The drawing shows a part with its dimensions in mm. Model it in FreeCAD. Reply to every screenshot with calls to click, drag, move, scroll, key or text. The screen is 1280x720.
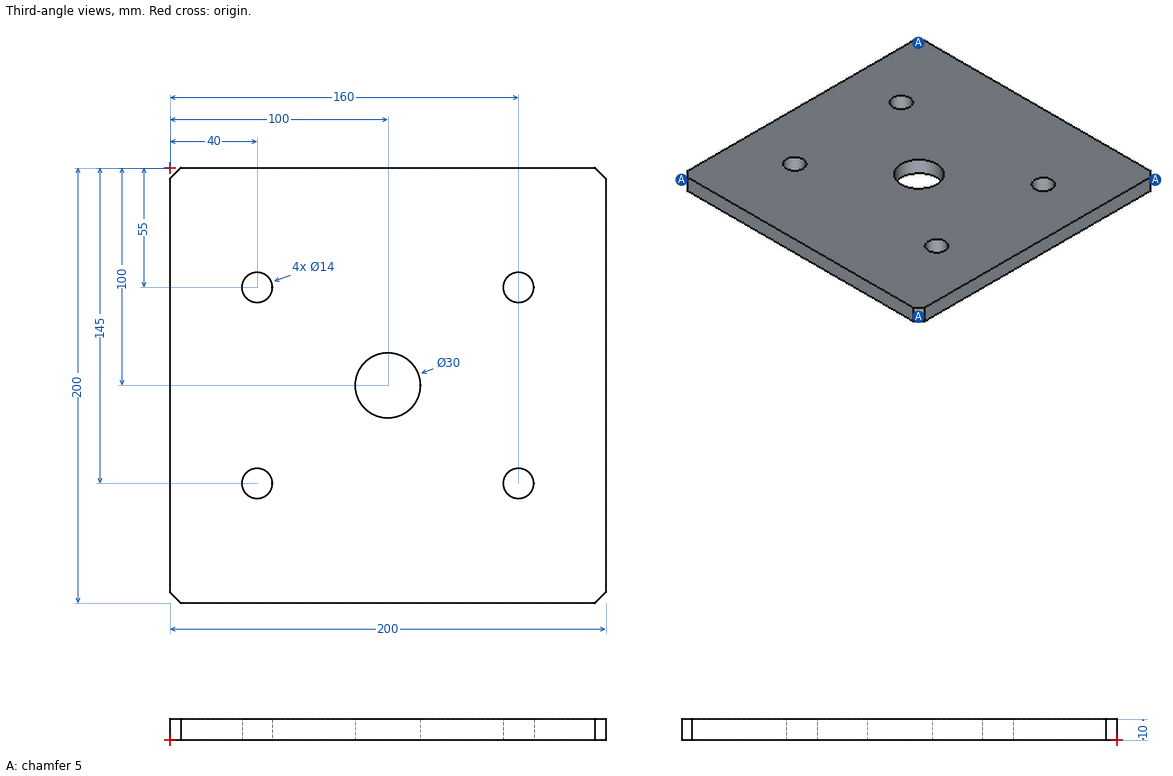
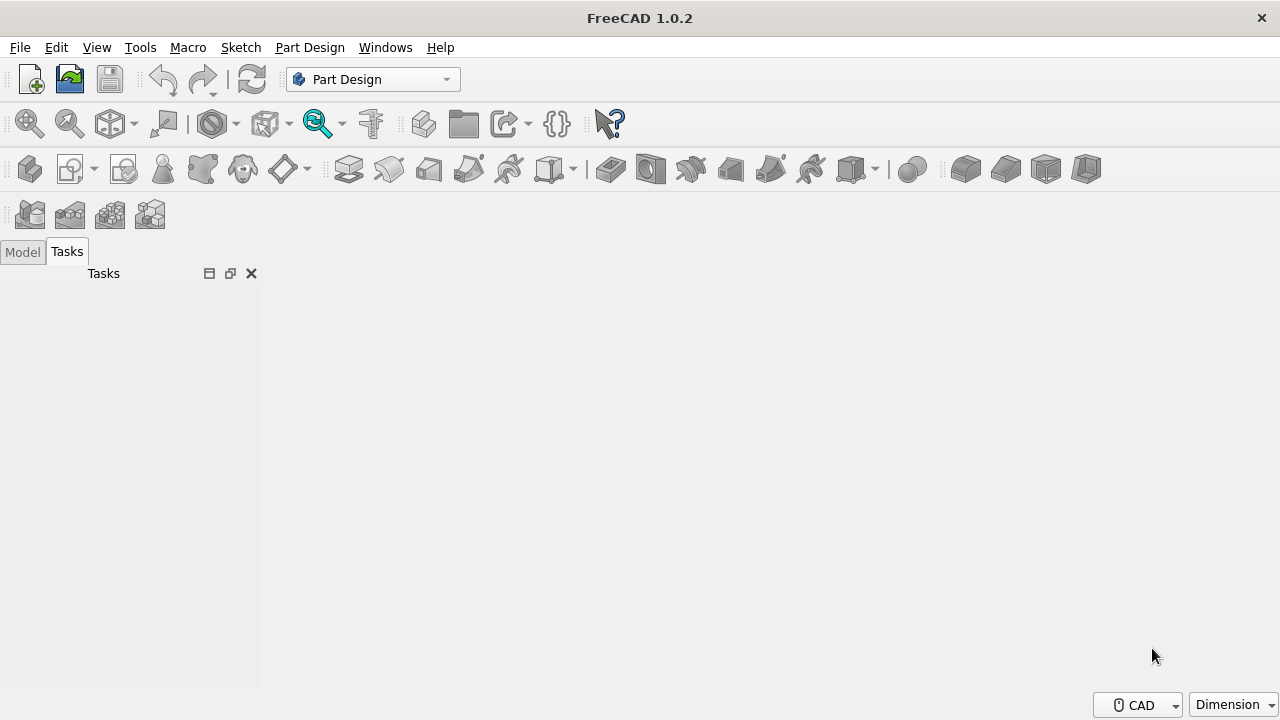
click(30, 80)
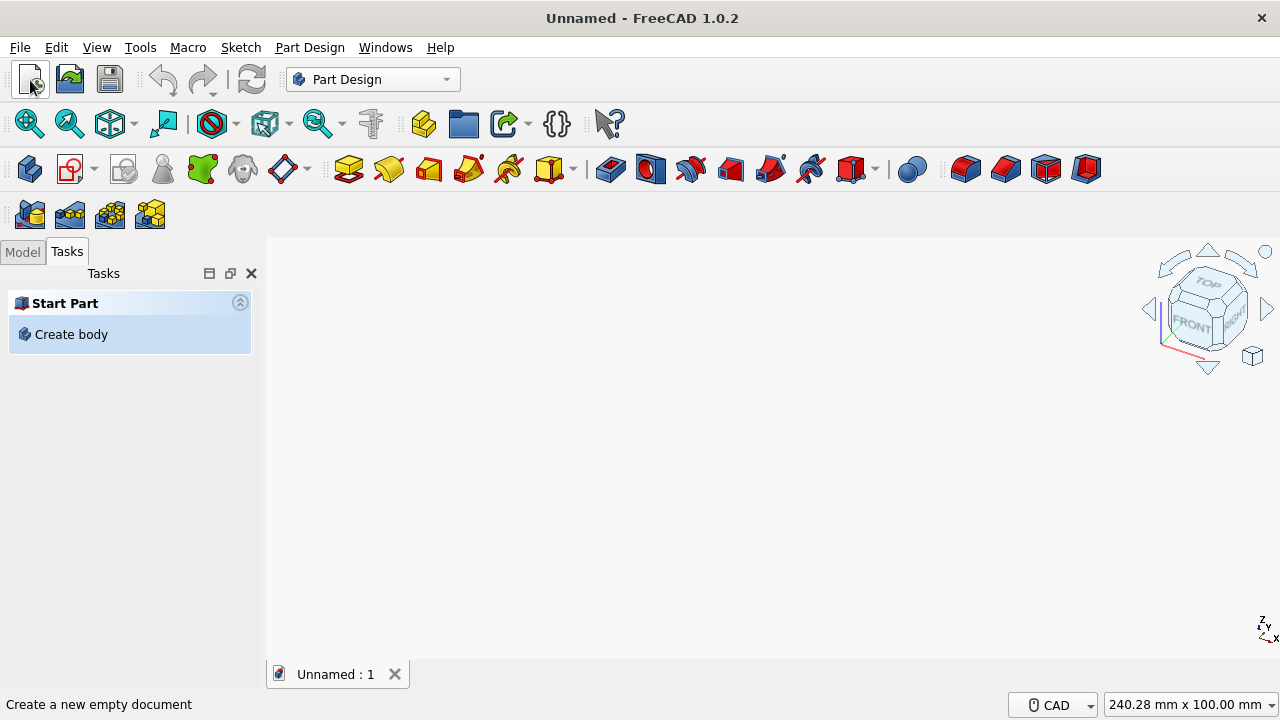
click(70, 170)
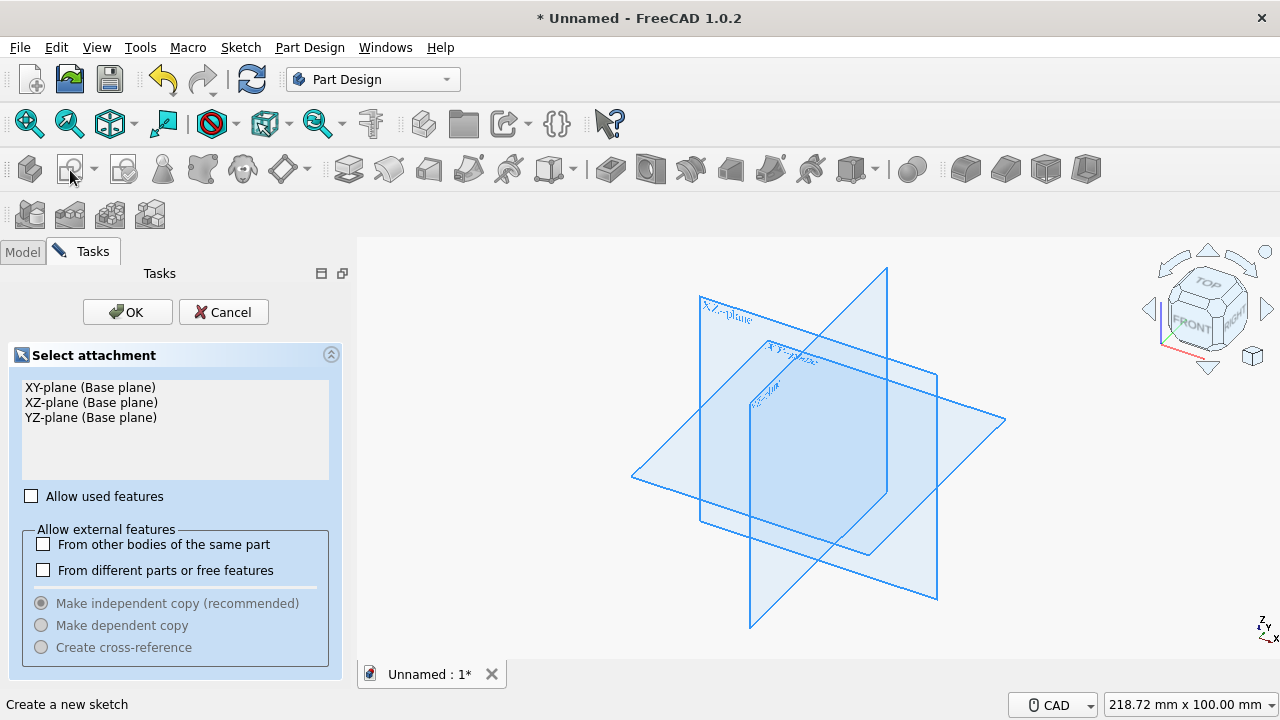
click(82, 388)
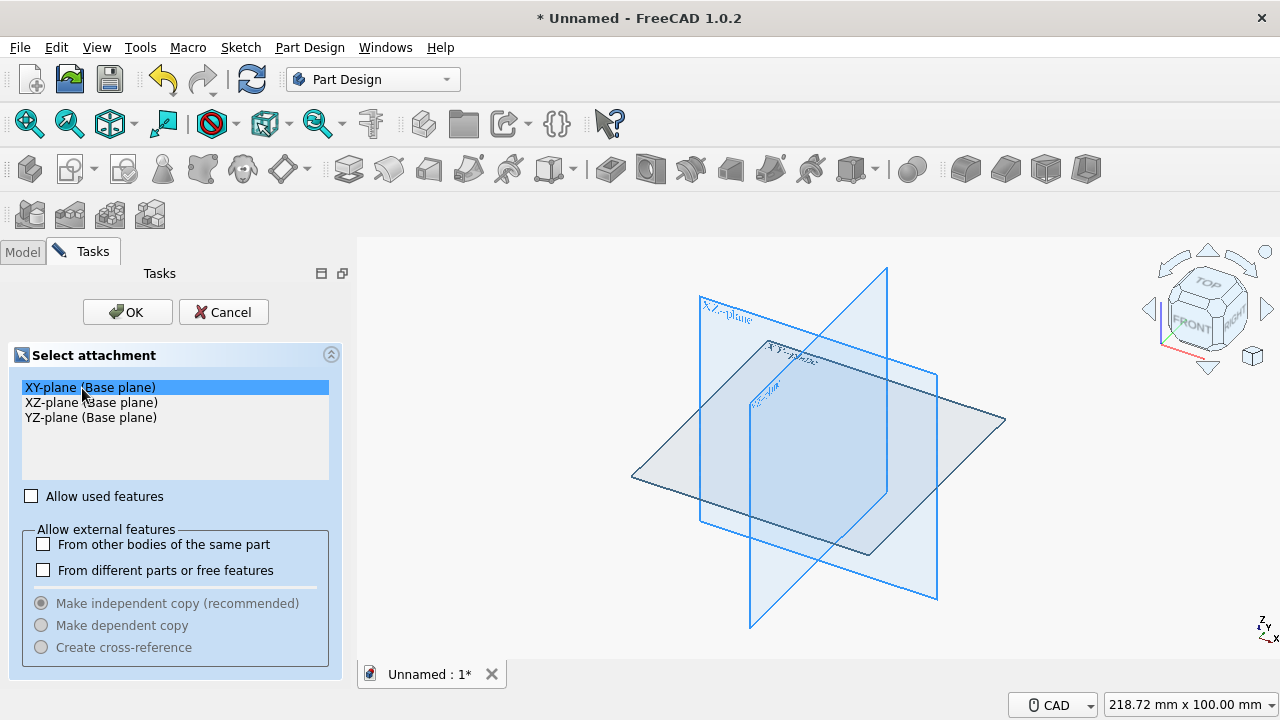
click(128, 312)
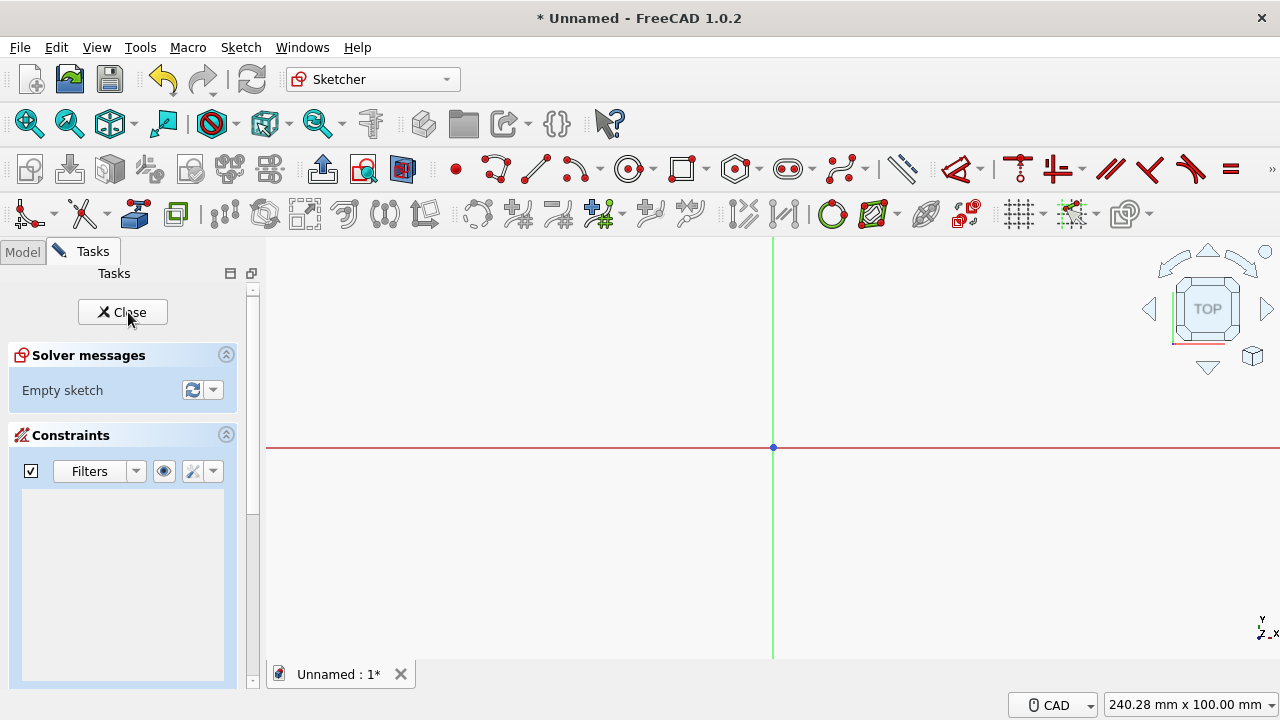
scroll(493, 266, down, 6)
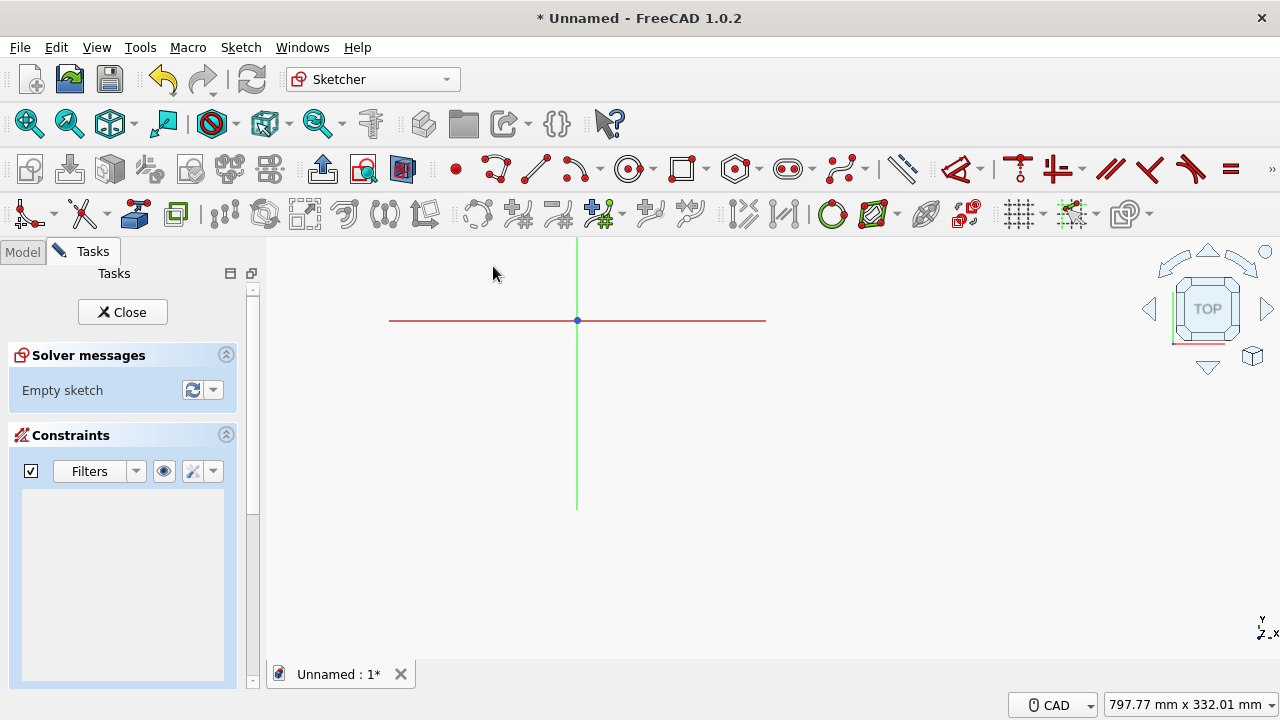
click(682, 170)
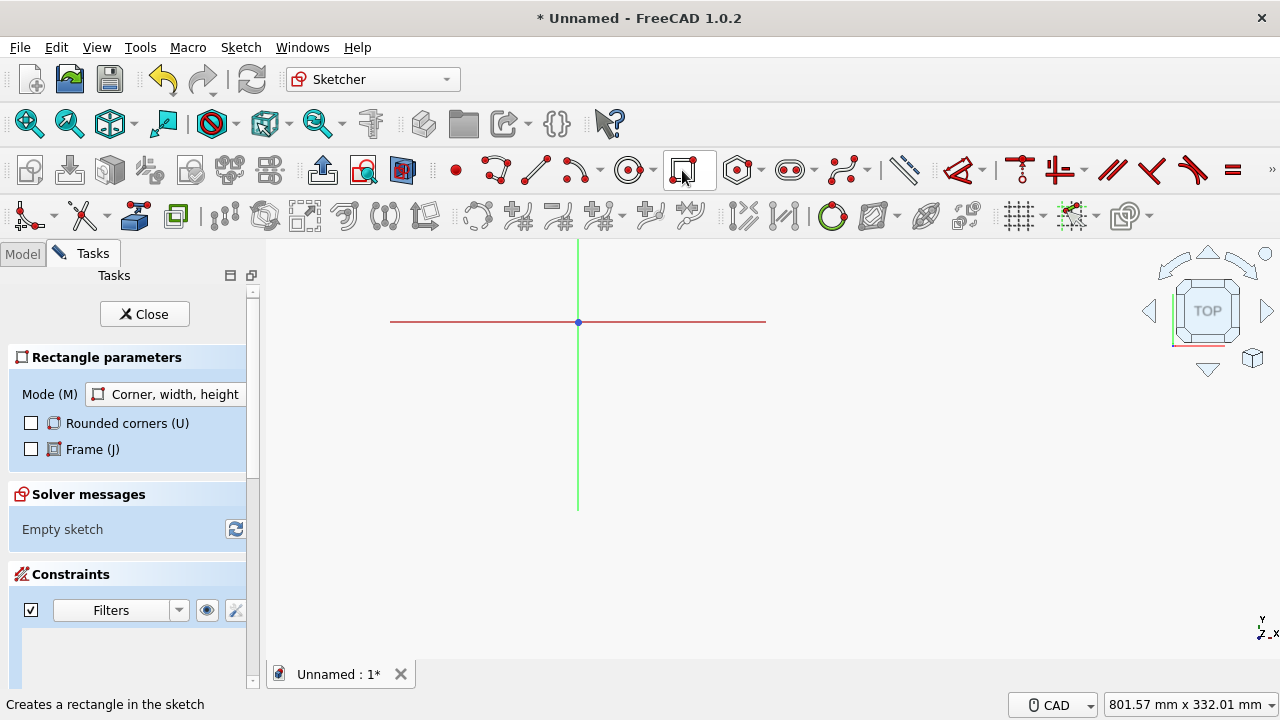
click(578, 322)
click(831, 575)
key(Escape)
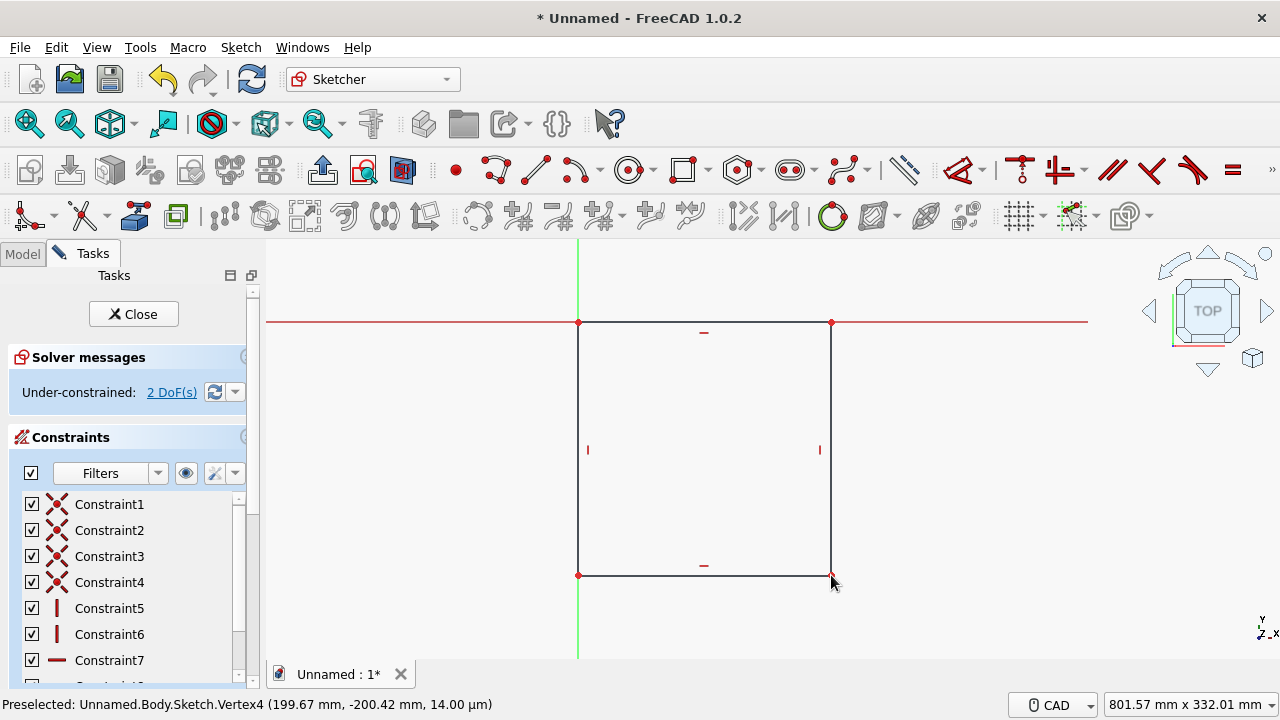
click(958, 170)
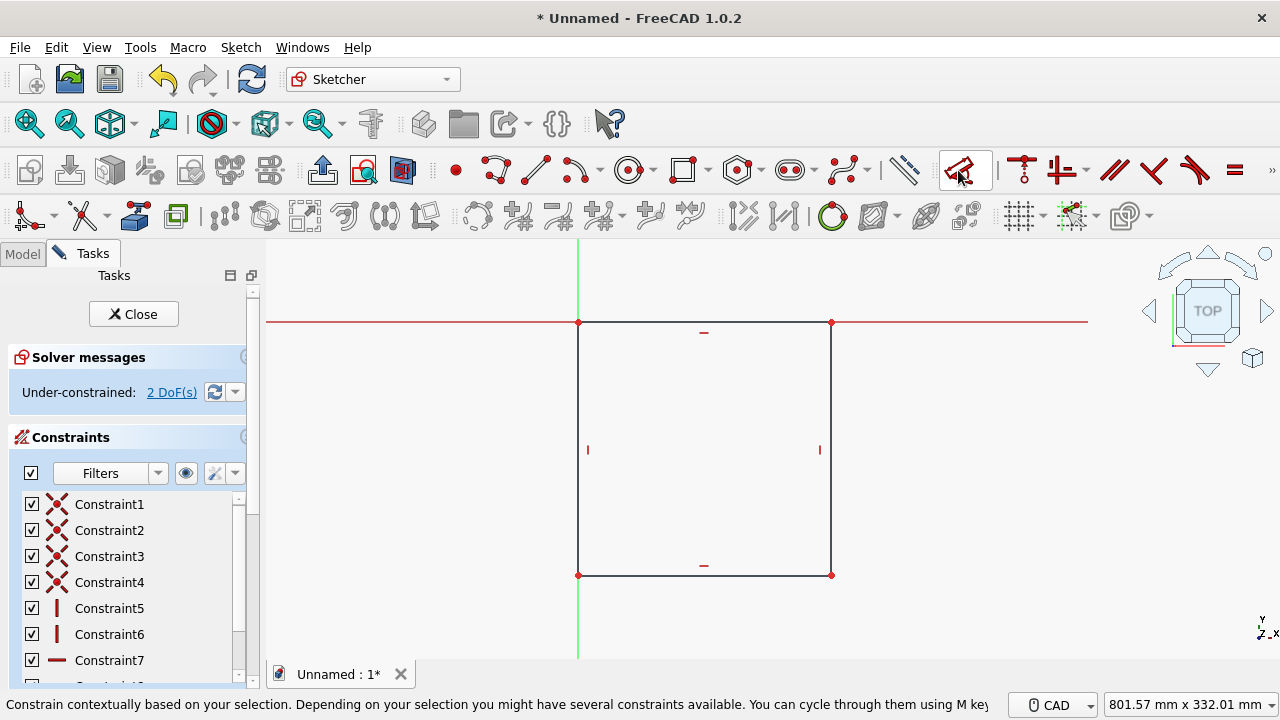
click(578, 399)
click(544, 449)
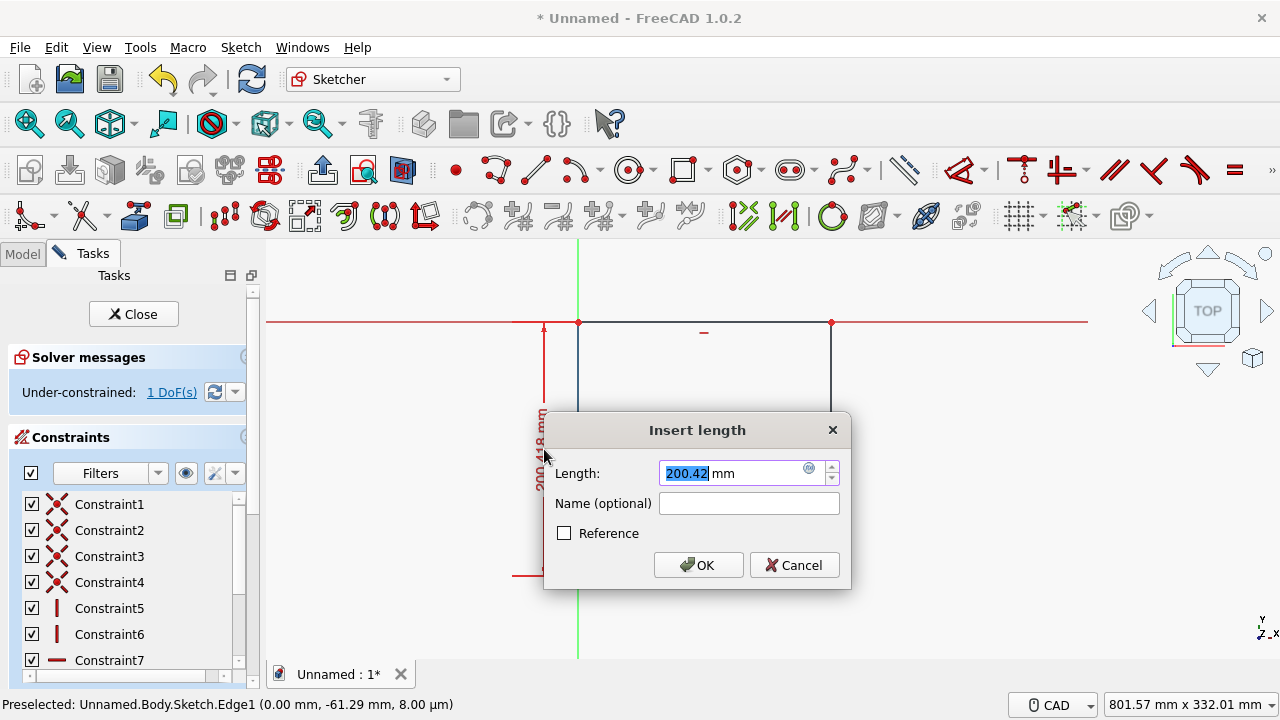
text(200)
key(Return)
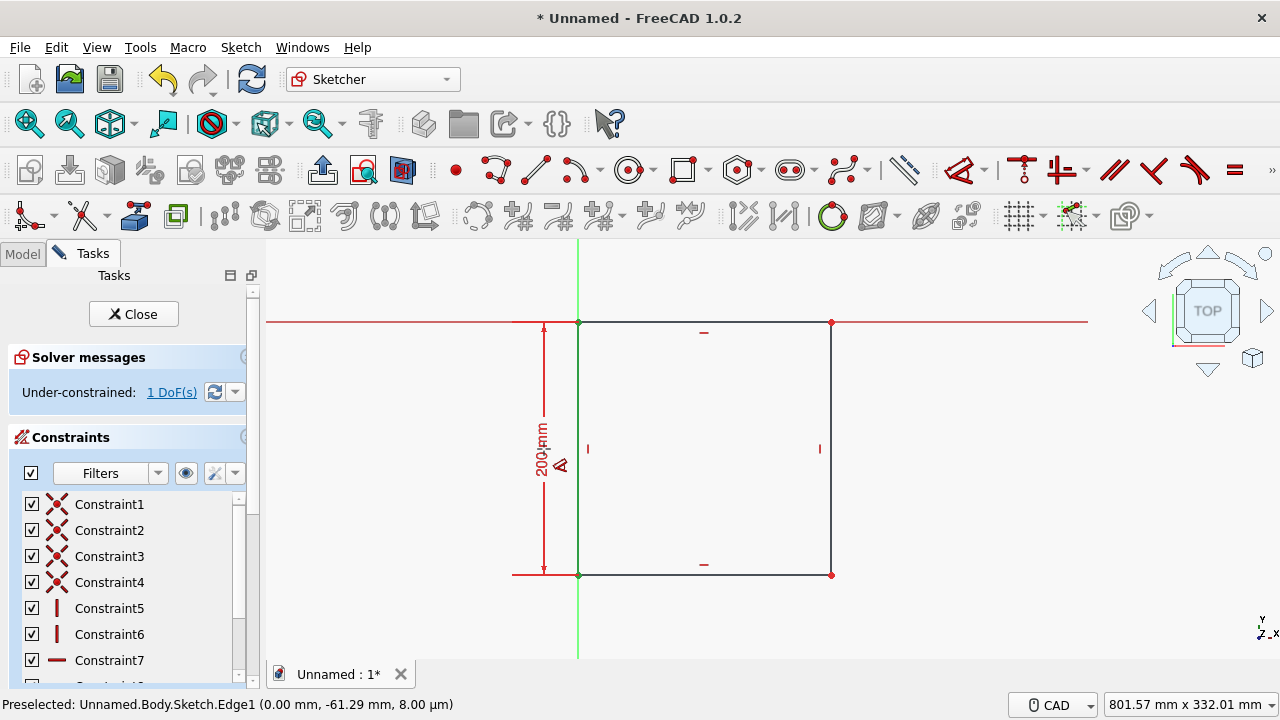
click(654, 575)
click(705, 609)